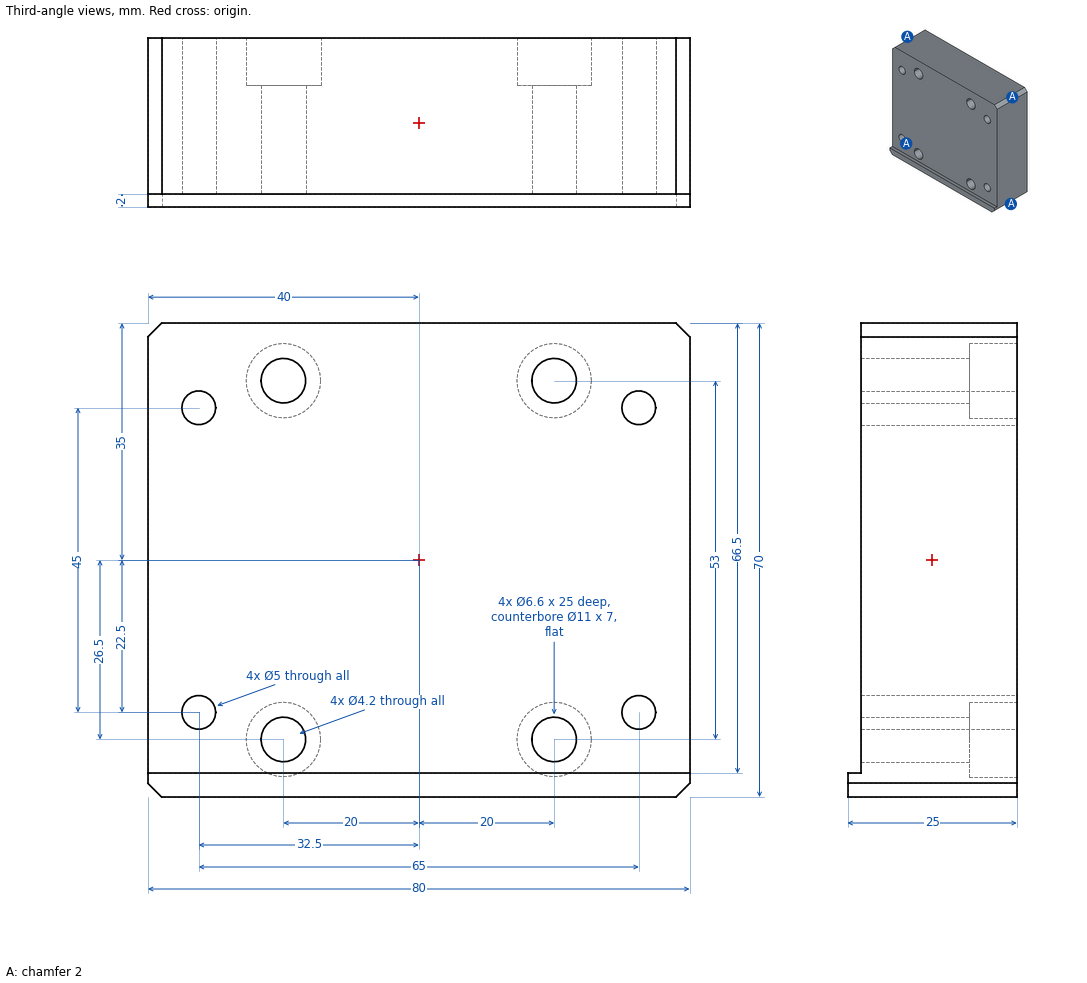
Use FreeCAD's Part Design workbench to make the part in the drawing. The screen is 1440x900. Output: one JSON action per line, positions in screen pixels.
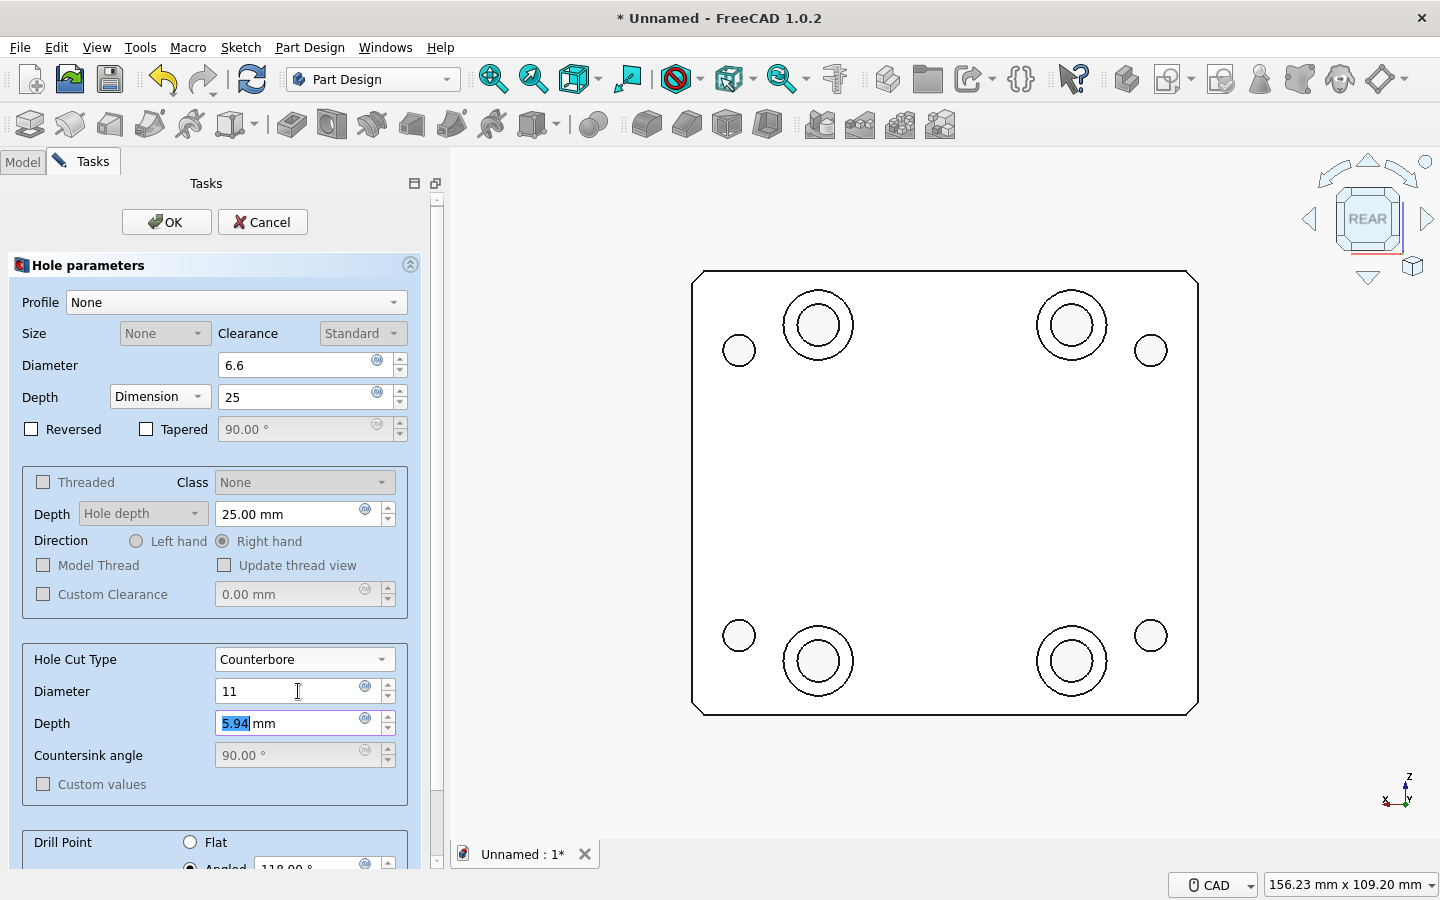
{"action": "type", "text": "7"}
{"action": "key", "text": "Tab"}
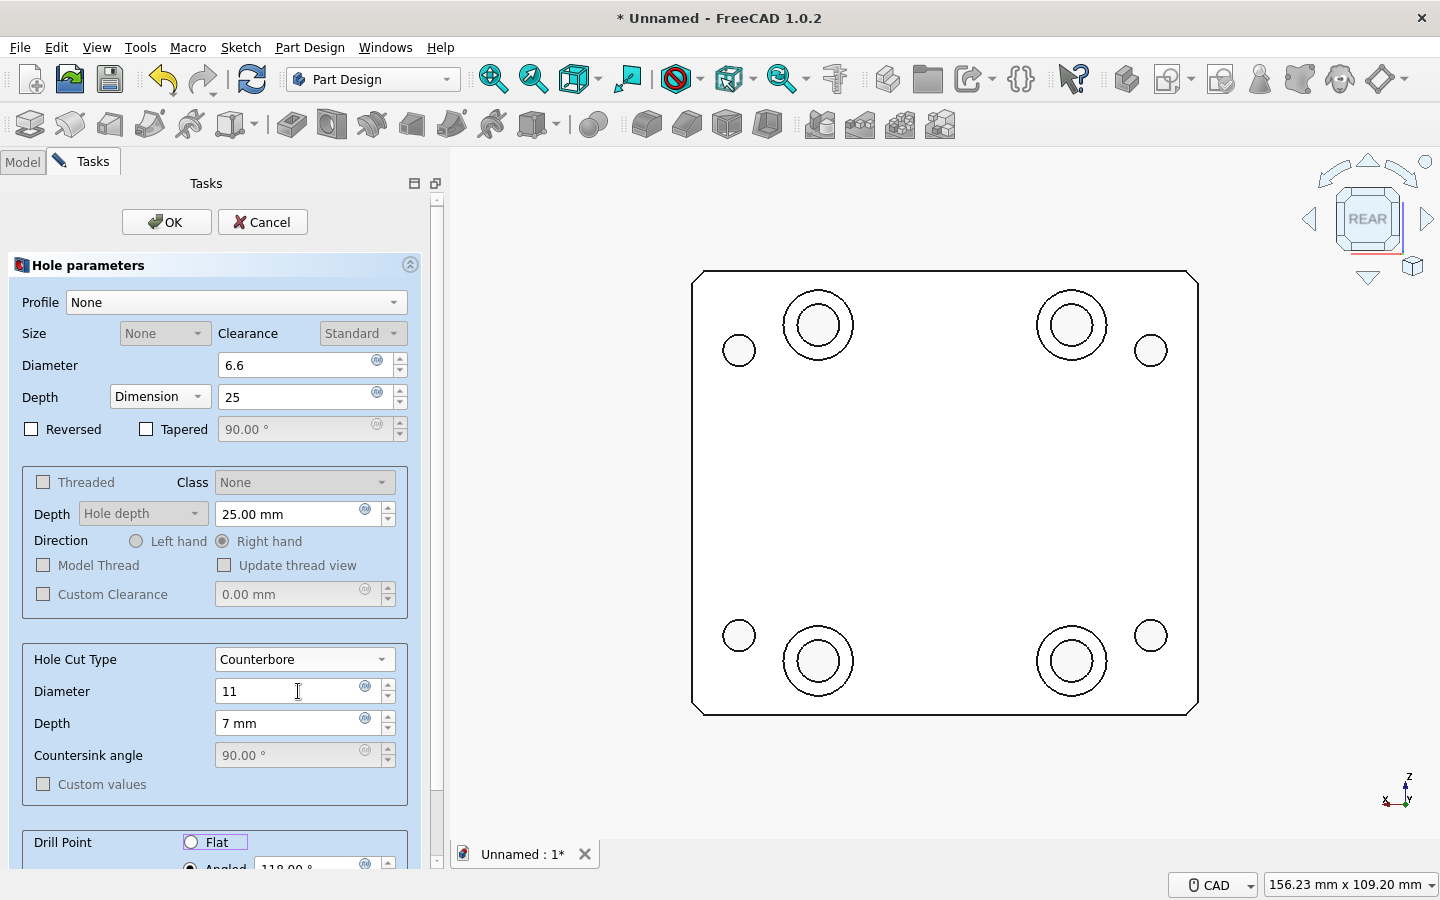
{"action": "left_click", "coordinate": [191, 842]}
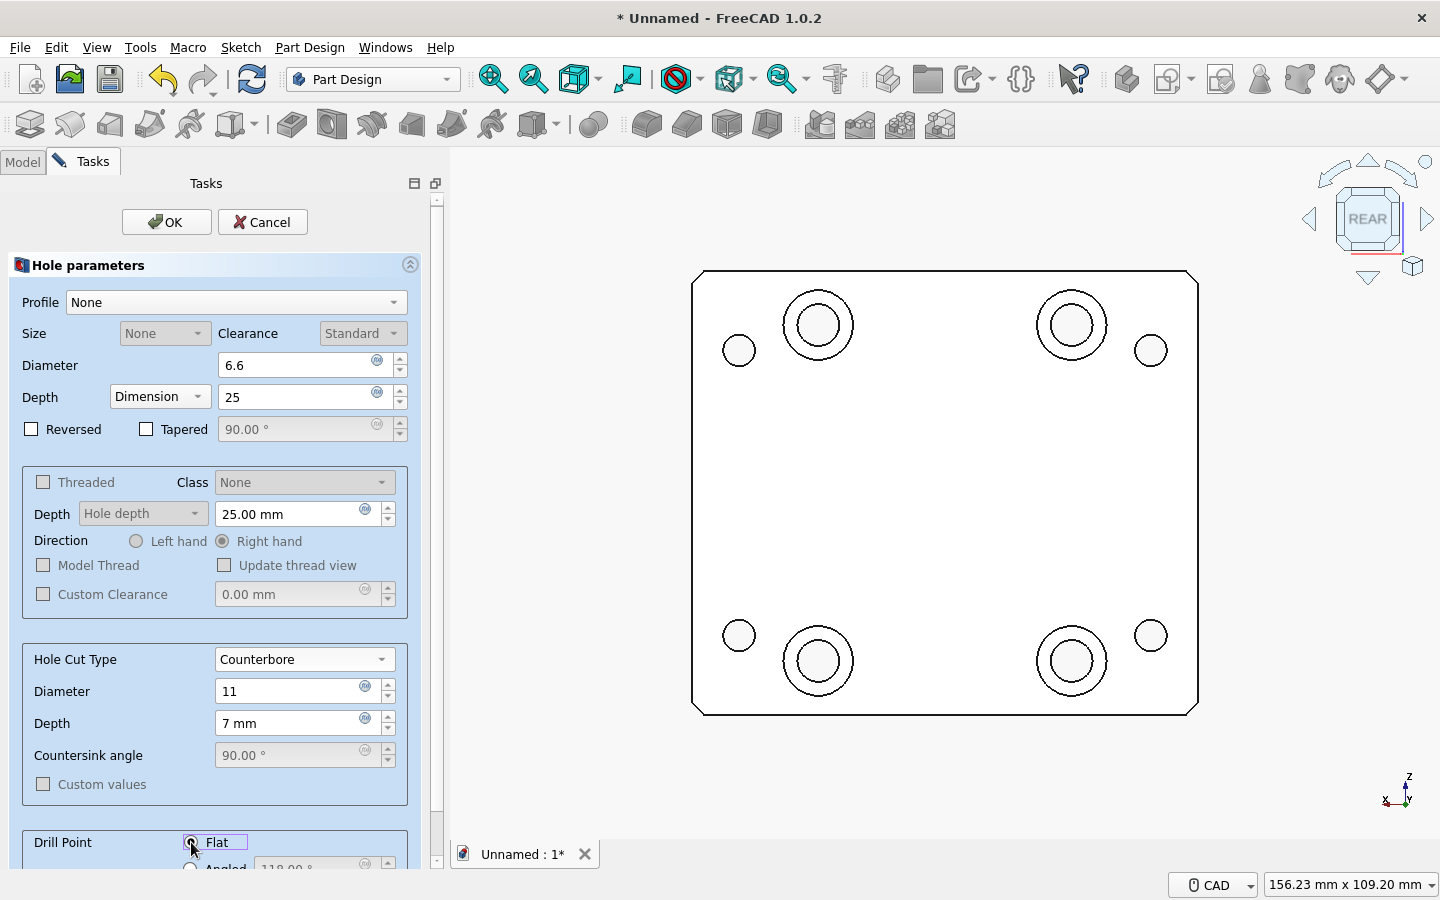
{"action": "left_click", "coordinate": [167, 222]}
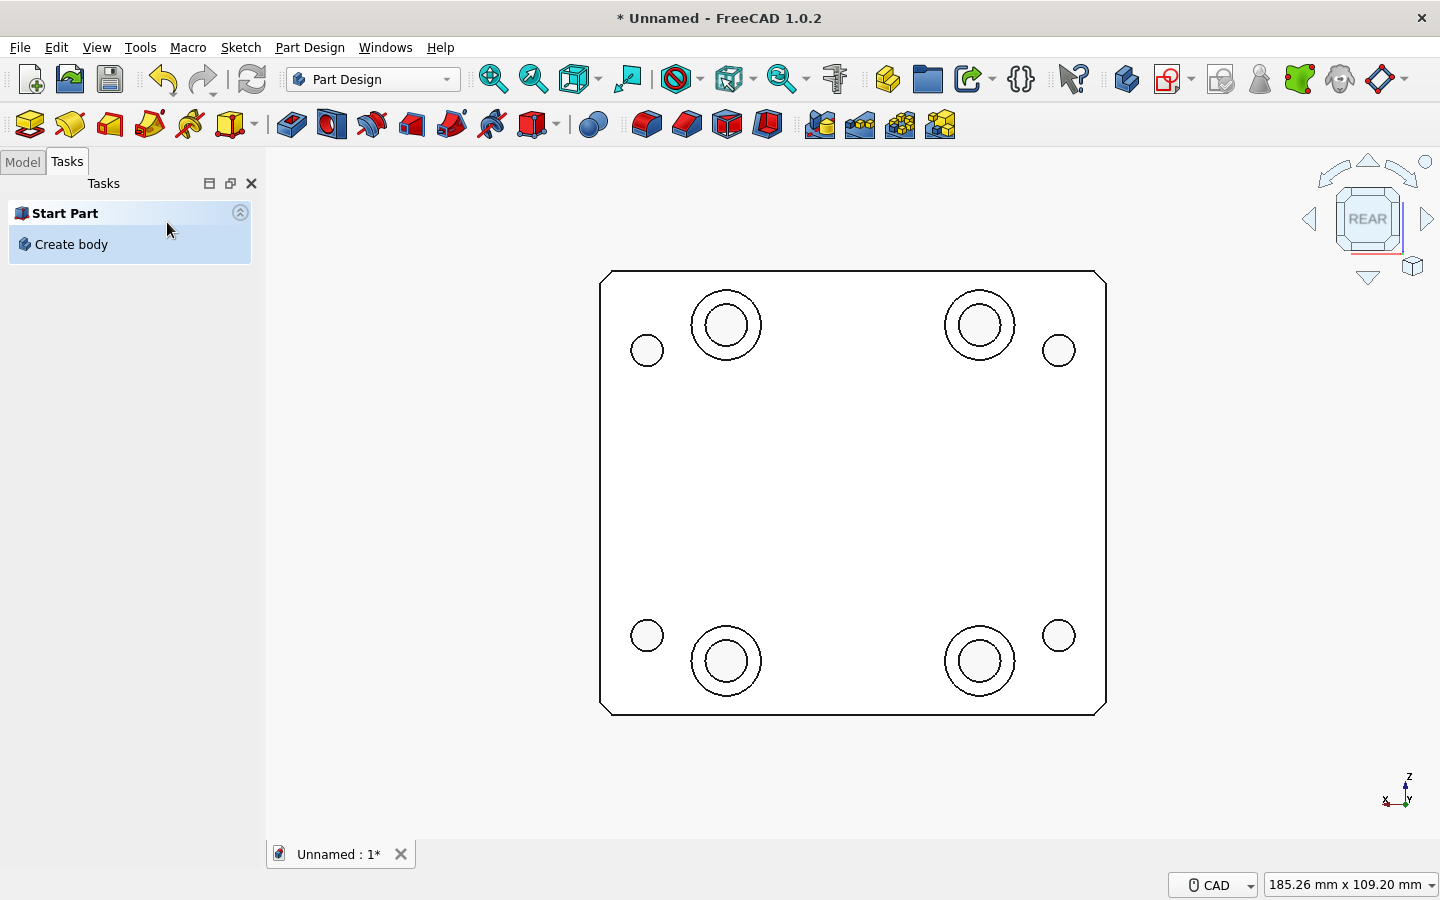
{"action": "key", "text": "0"}